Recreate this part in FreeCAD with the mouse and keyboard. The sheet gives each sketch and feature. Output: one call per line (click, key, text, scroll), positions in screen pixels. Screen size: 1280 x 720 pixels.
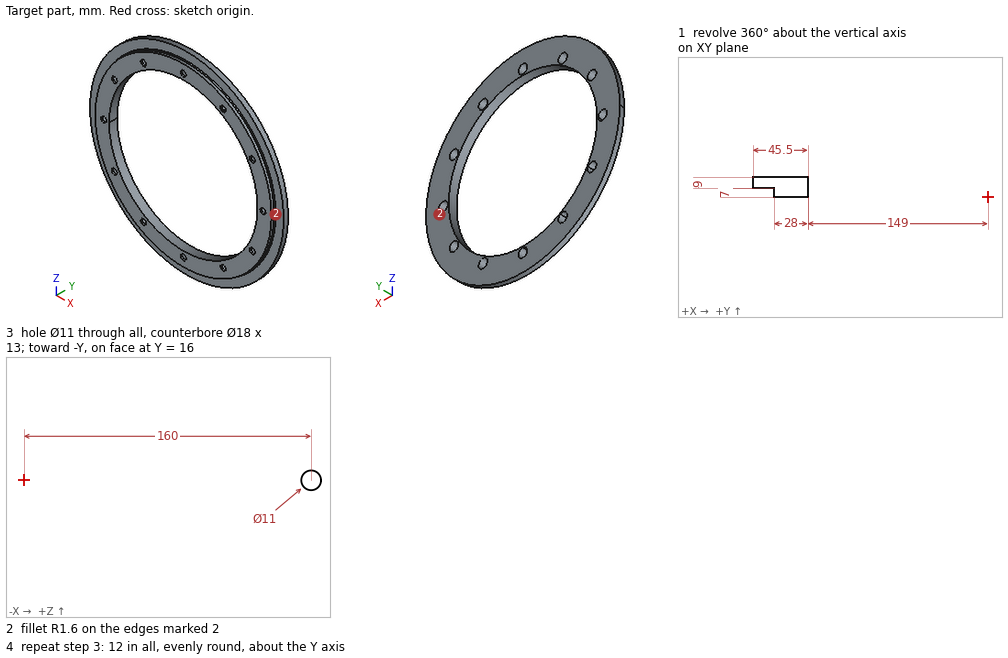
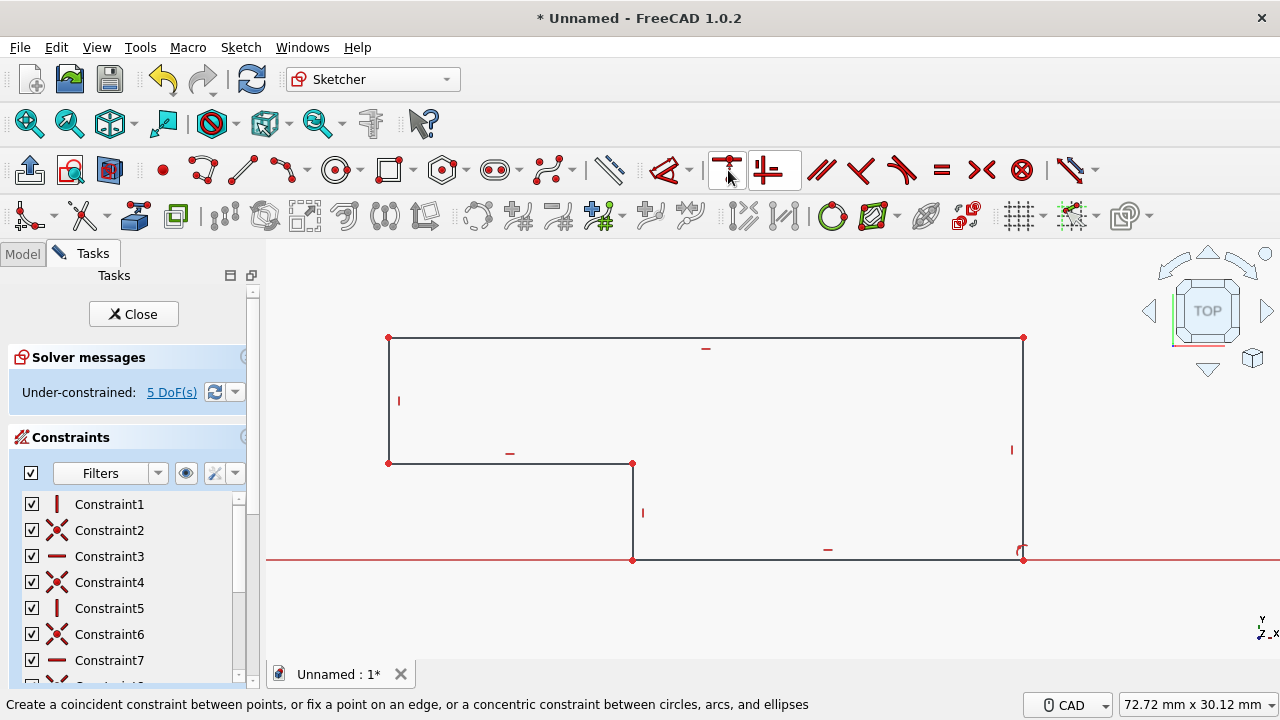
click(664, 170)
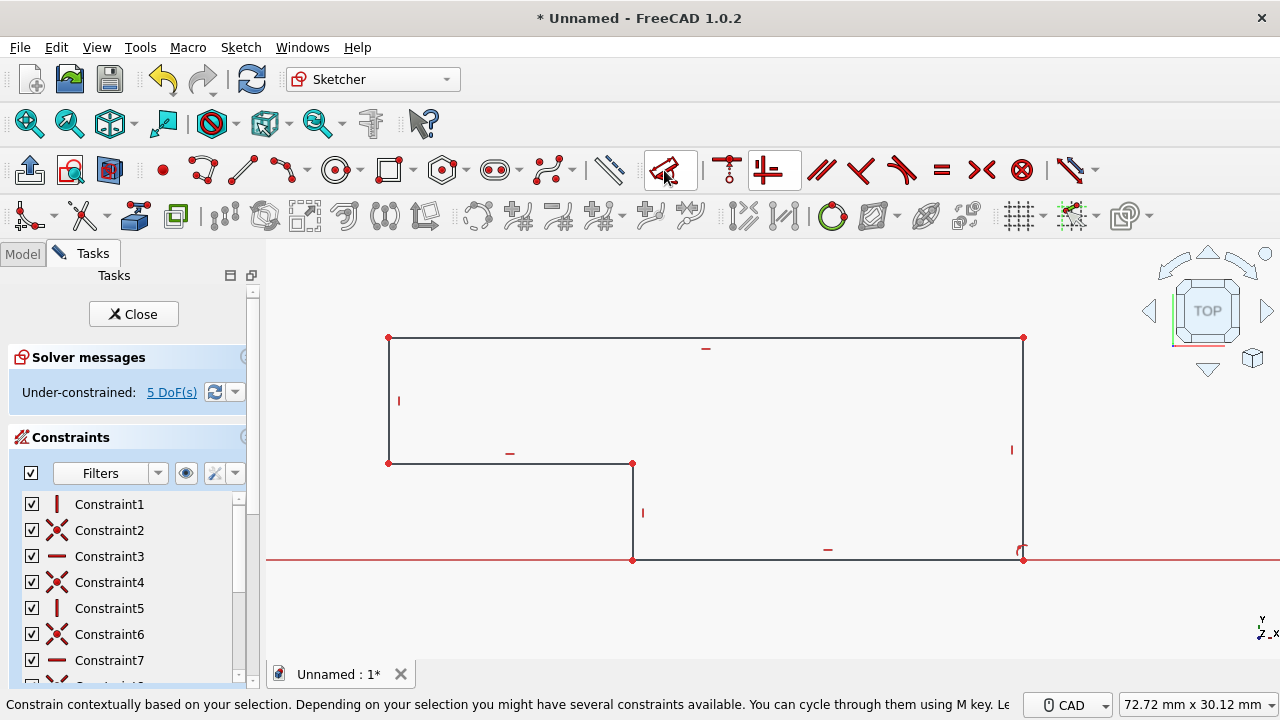
click(389, 376)
click(355, 401)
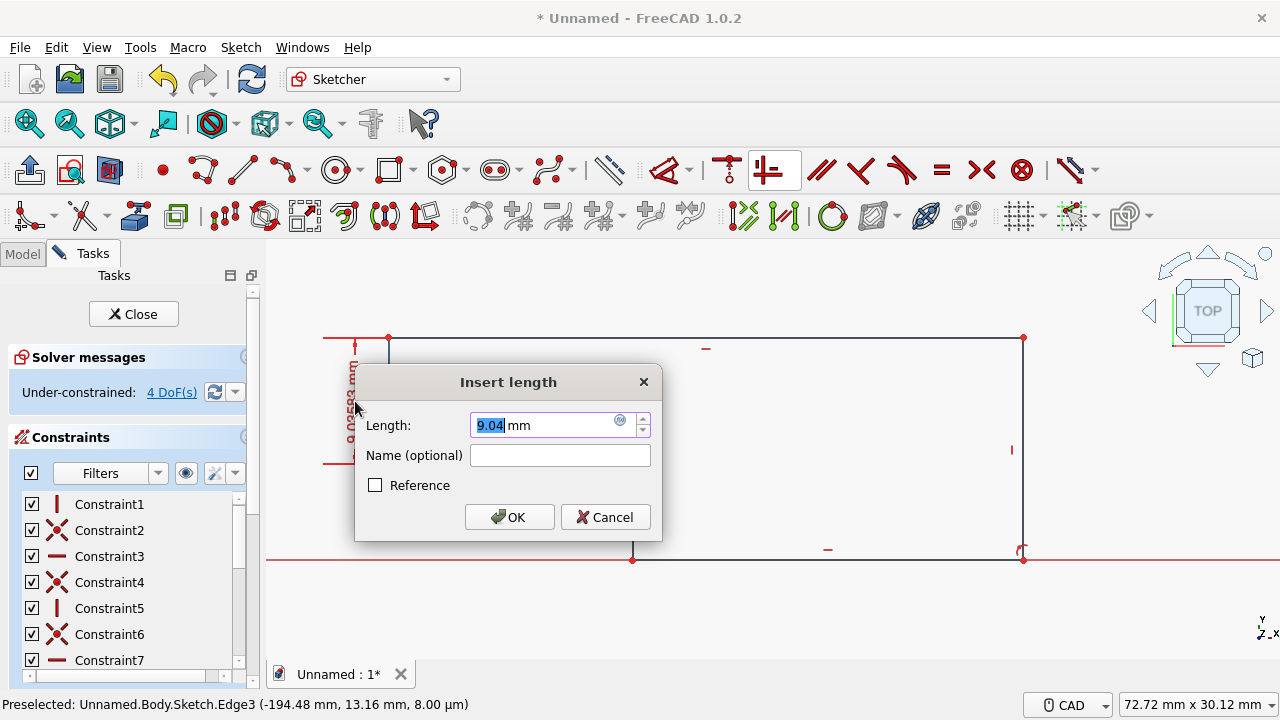
text(9)
key(Return)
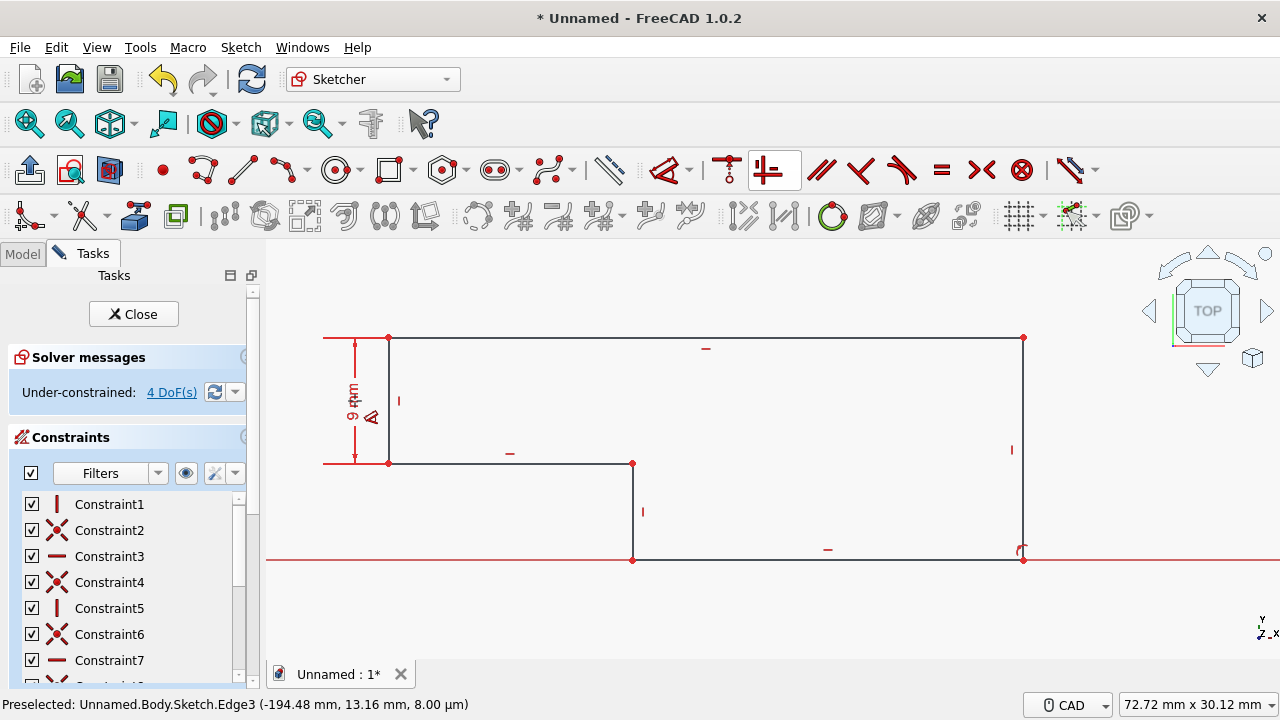
click(633, 493)
click(599, 512)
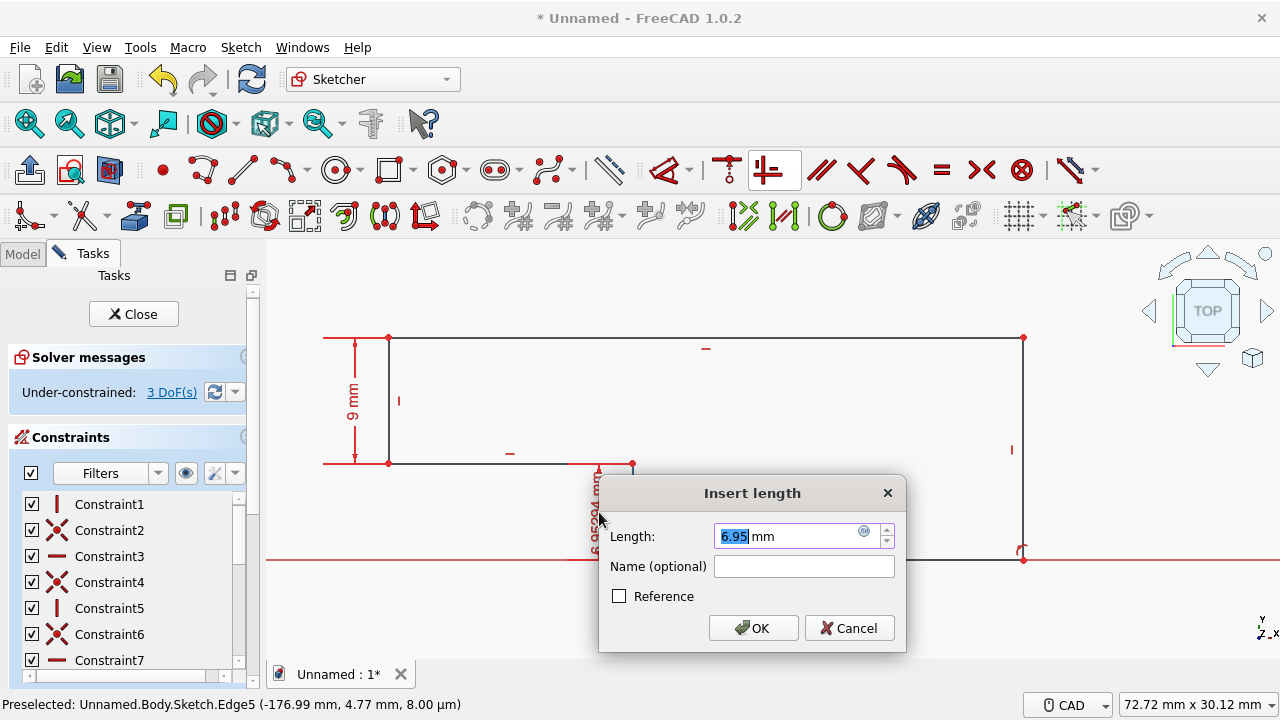
text(7)
key(Return)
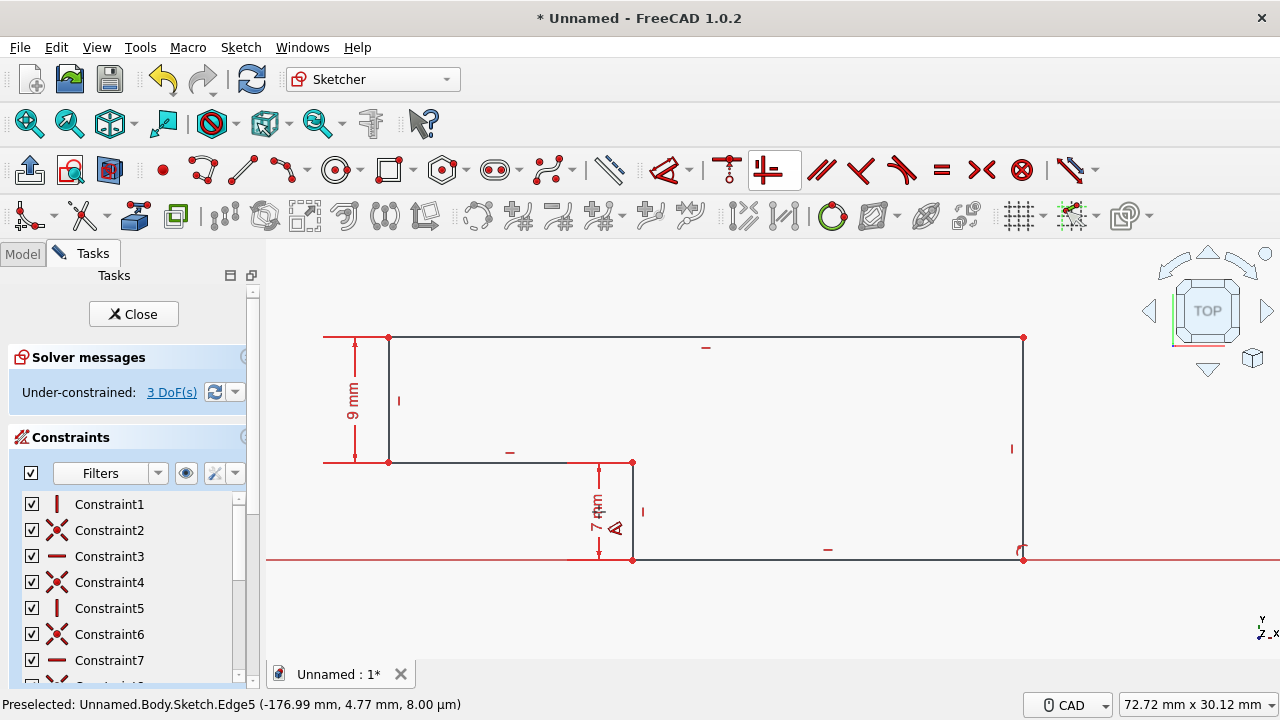
click(750, 560)
click(828, 594)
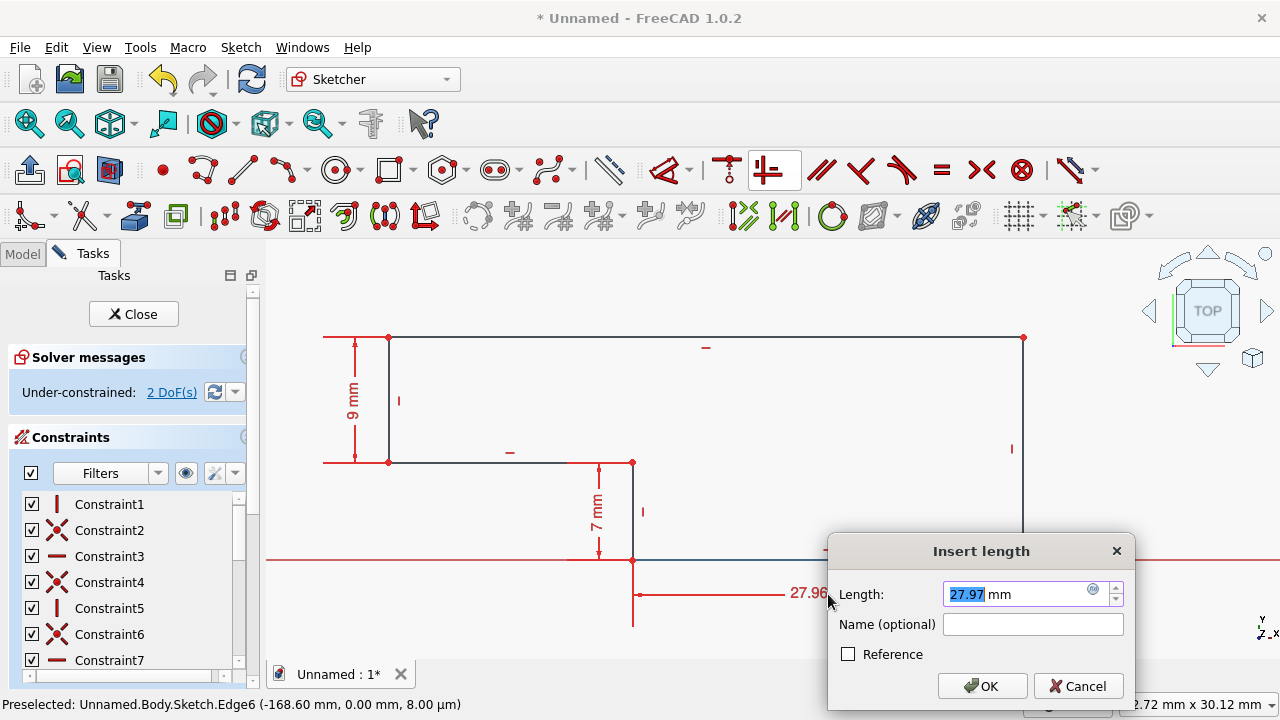
text(28)
key(Return)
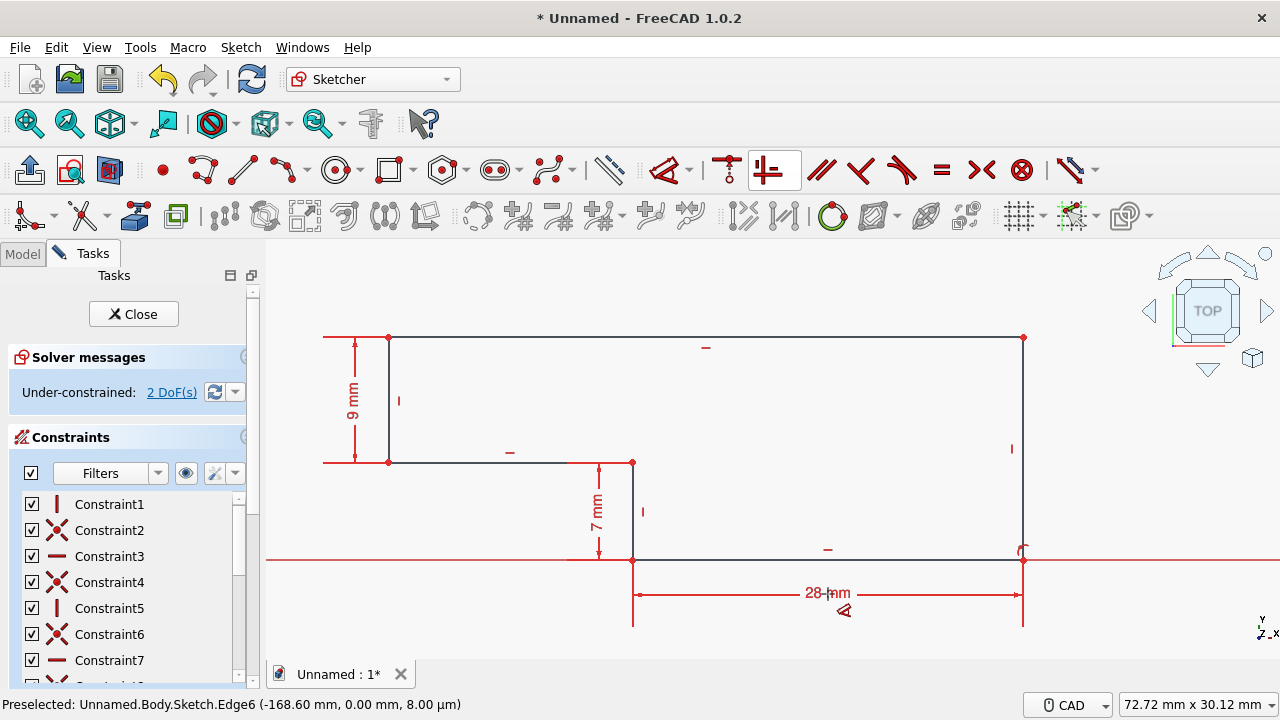
click(833, 337)
click(706, 303)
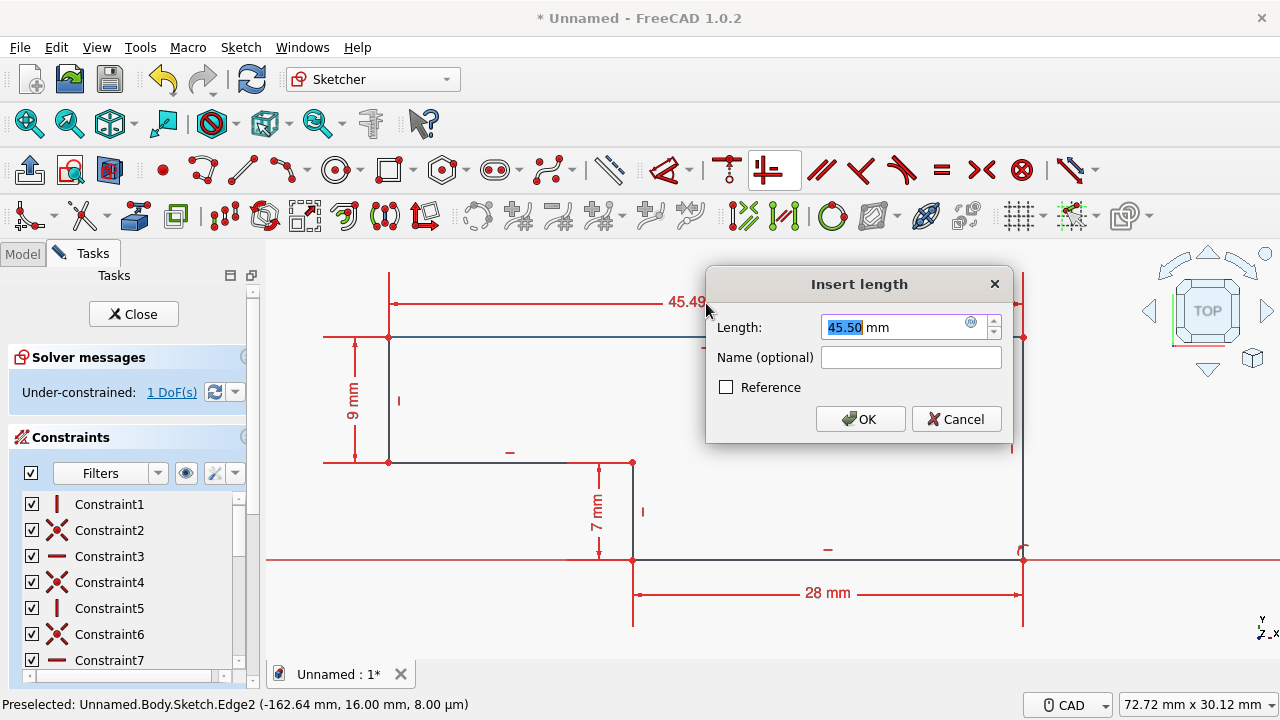
text(45.5)
key(Return)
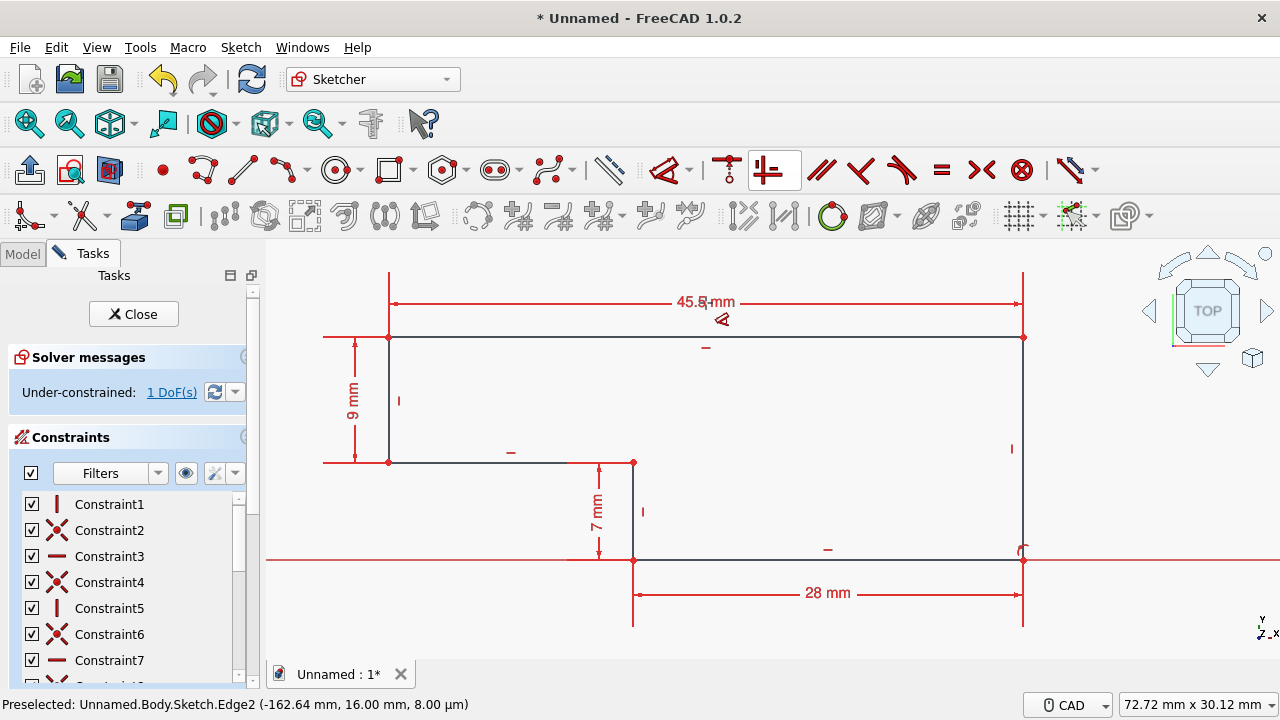
click(1023, 560)
click(1069, 594)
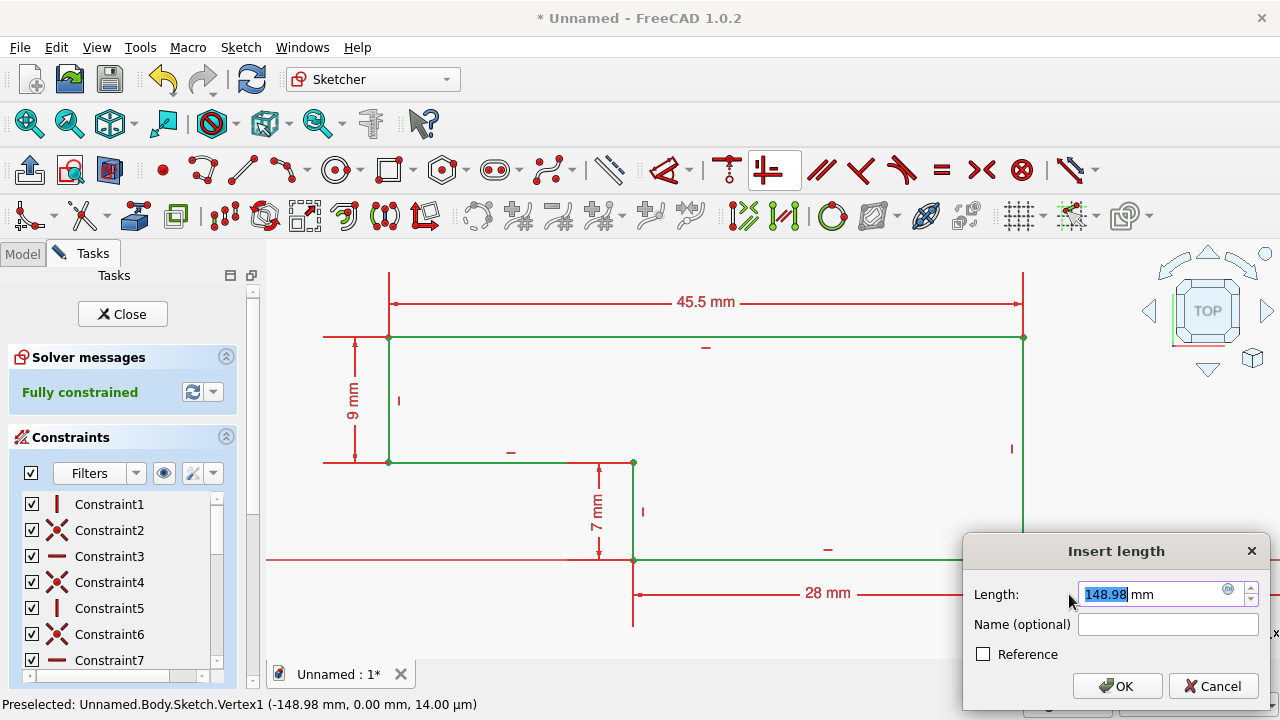
text(149)
key(Return)
key(Escape)